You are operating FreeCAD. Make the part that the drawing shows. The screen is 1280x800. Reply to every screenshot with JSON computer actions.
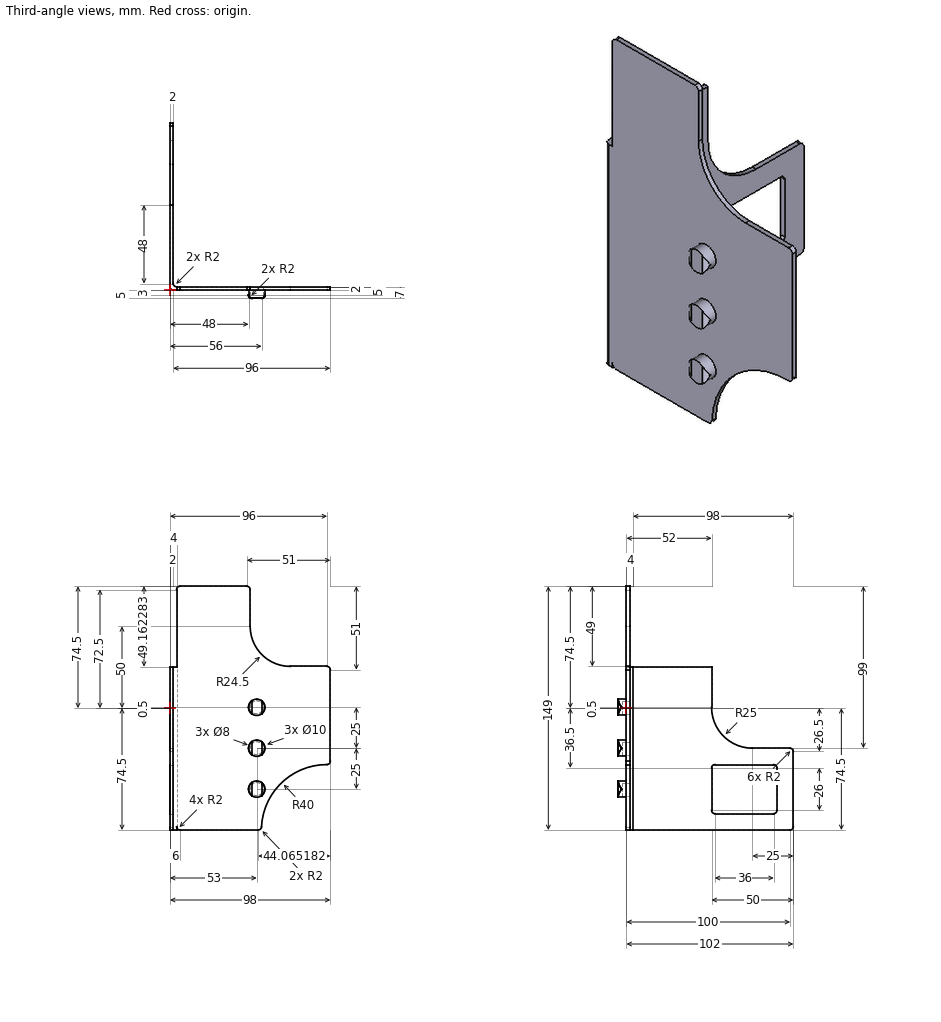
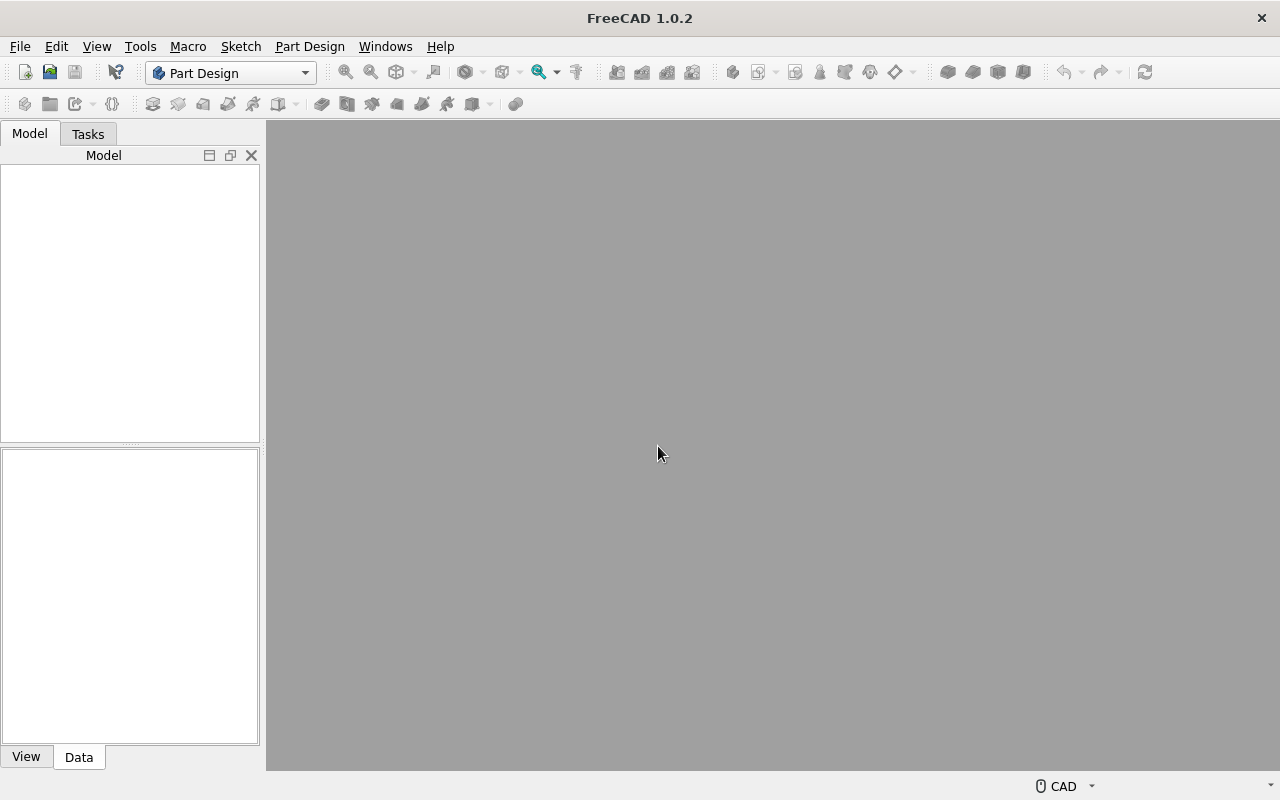
{"action": "key", "text": "ctrl+n"}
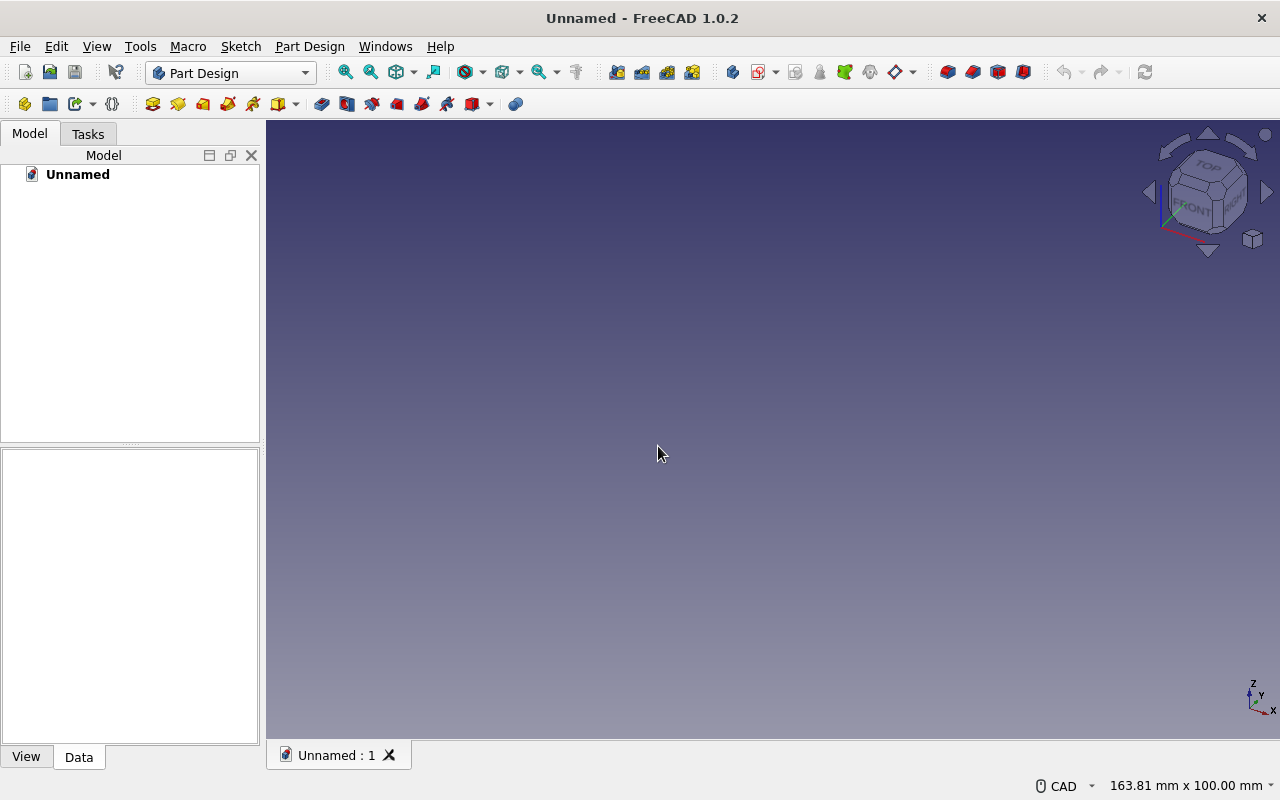
{"action": "left_click", "coordinate": [758, 72]}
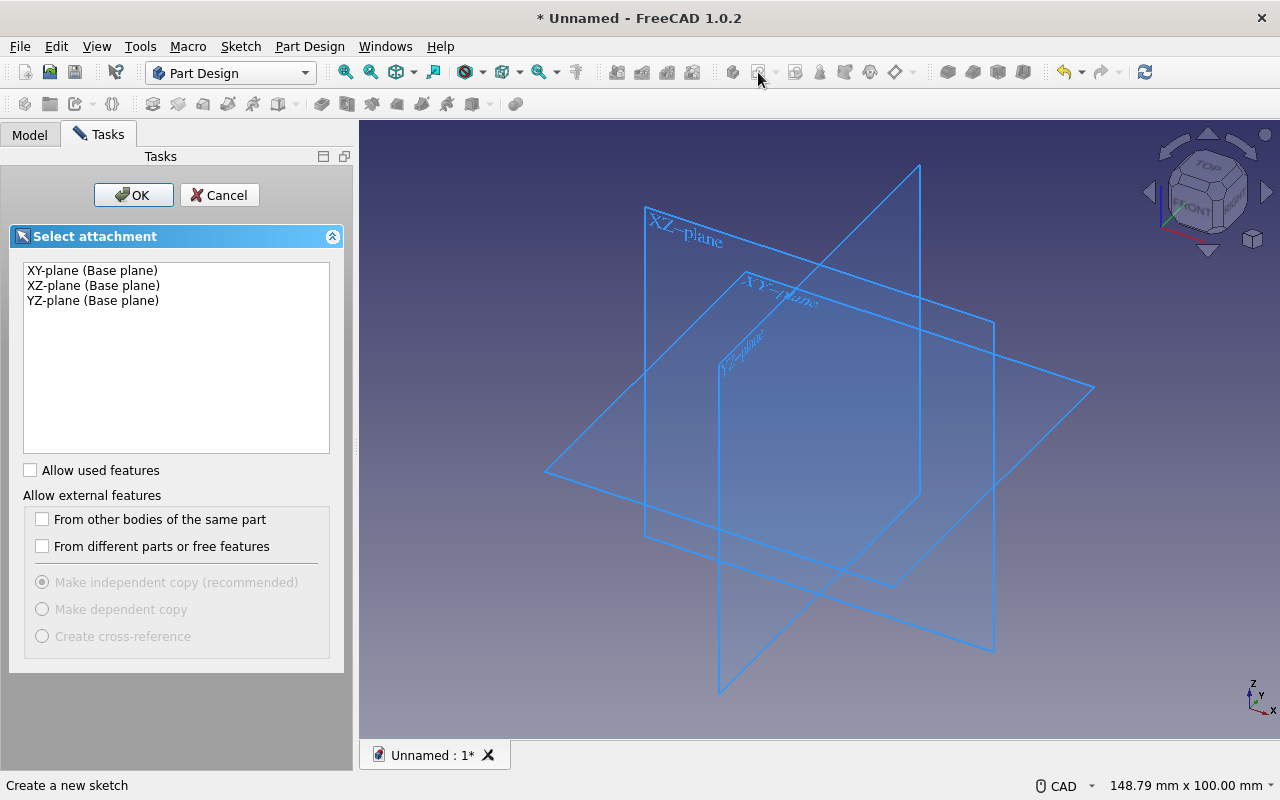
{"action": "left_click", "coordinate": [84, 270]}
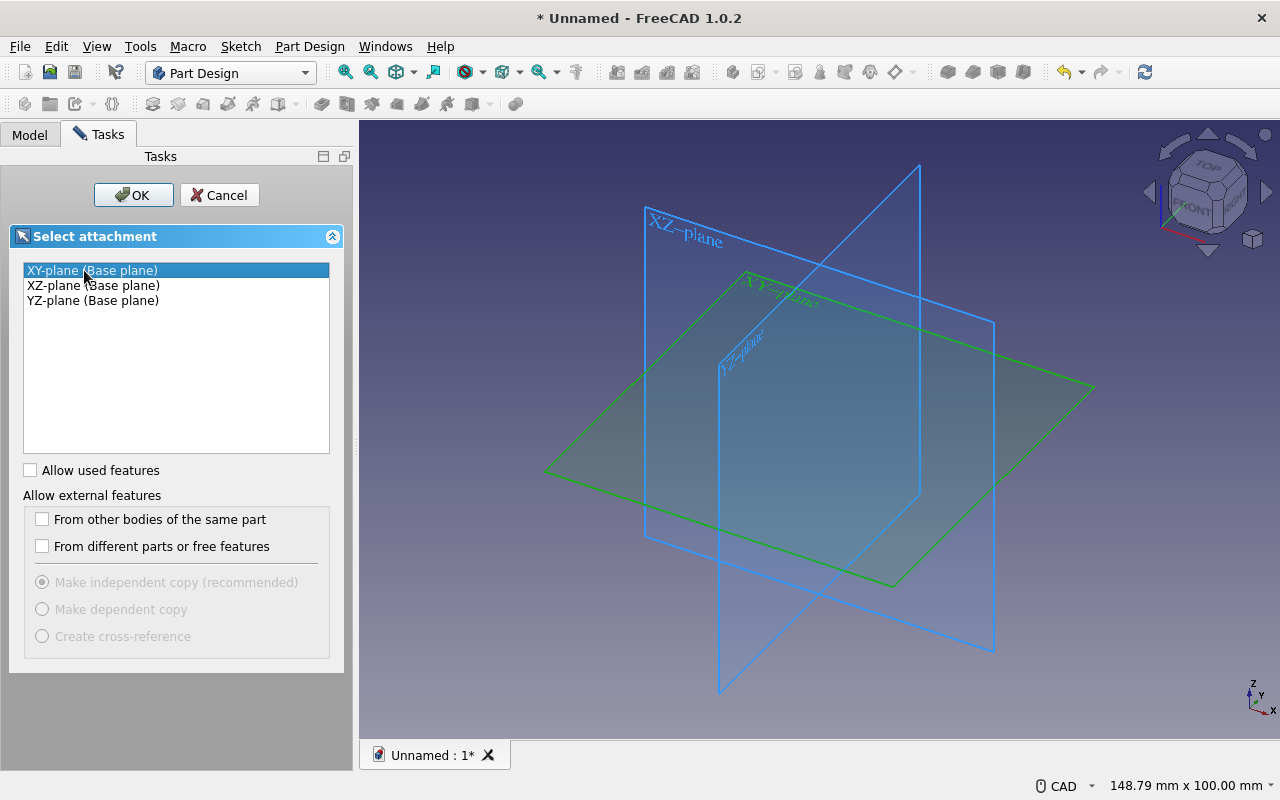
{"action": "left_click", "coordinate": [134, 195]}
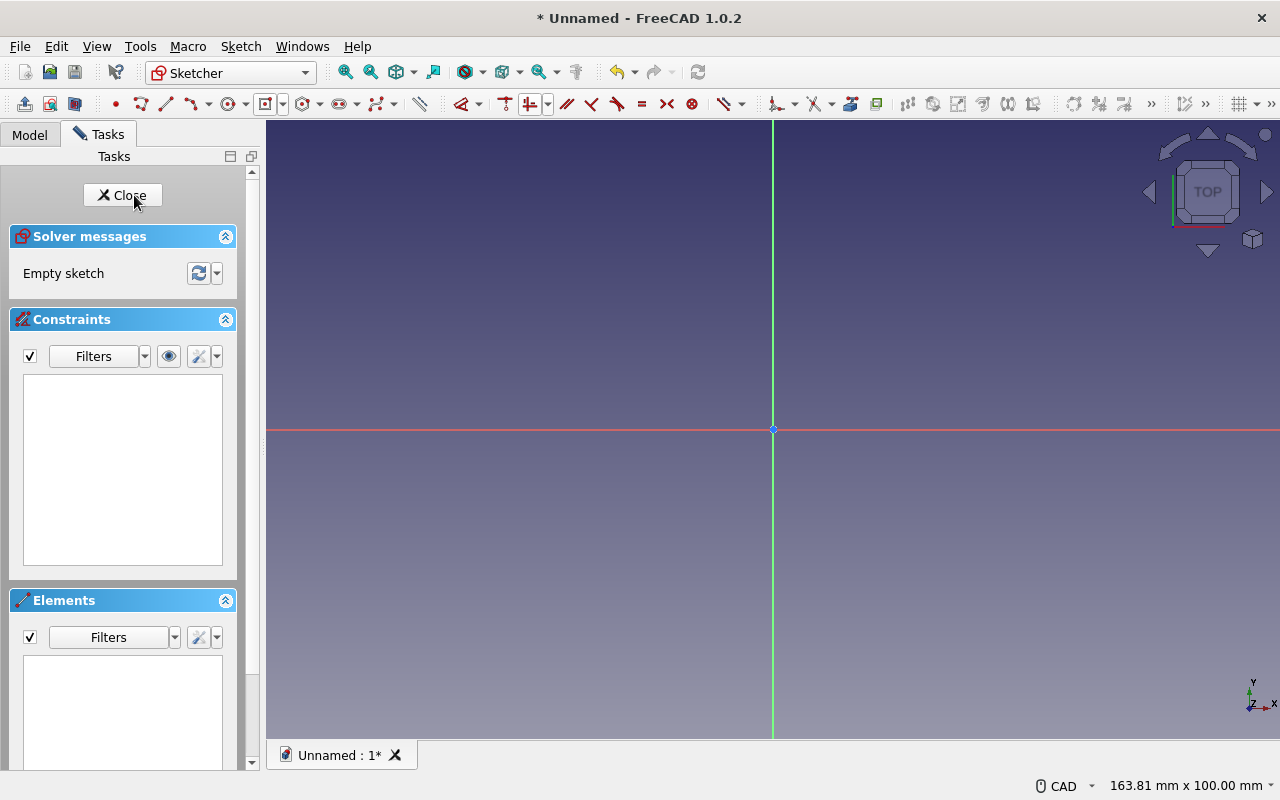
{"action": "scroll", "coordinate": [294, 711], "scroll_direction": "down", "scroll_amount": 2}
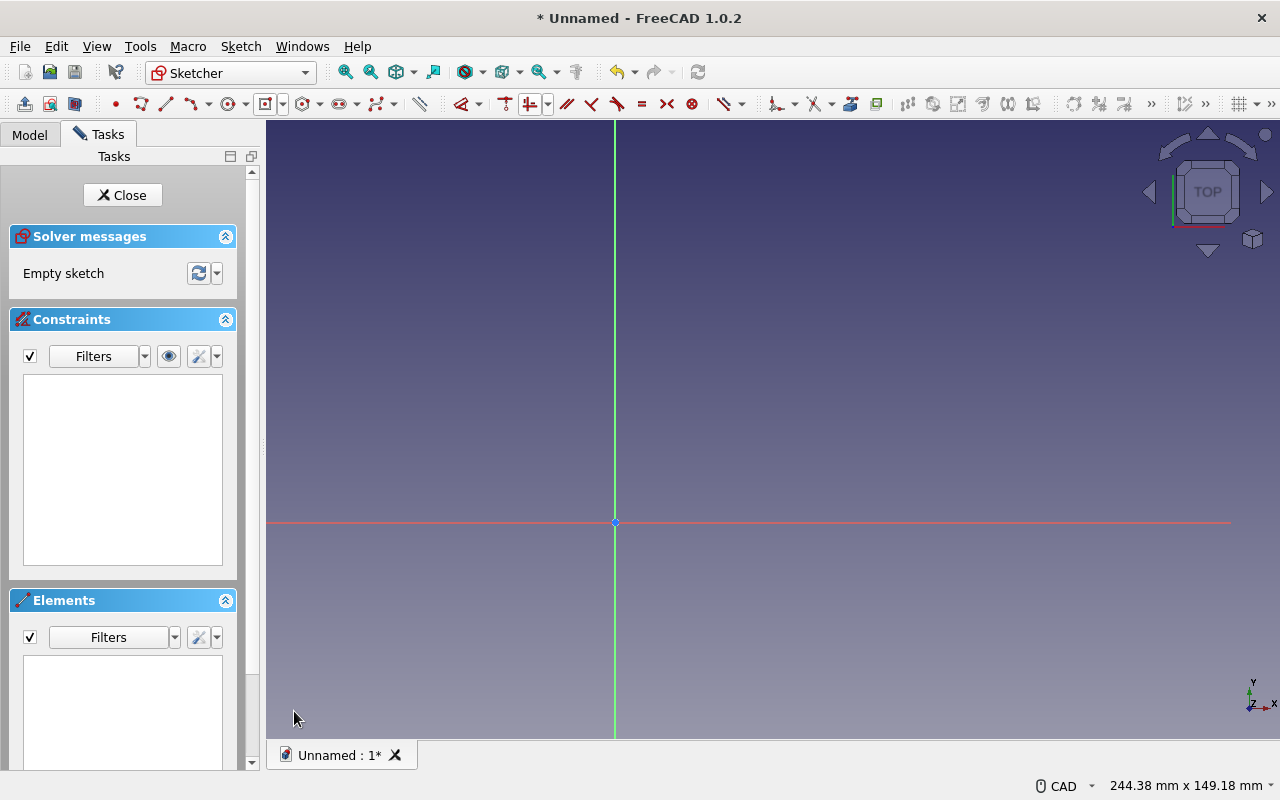
{"action": "scroll", "coordinate": [1050, 385], "scroll_direction": "up", "scroll_amount": 2}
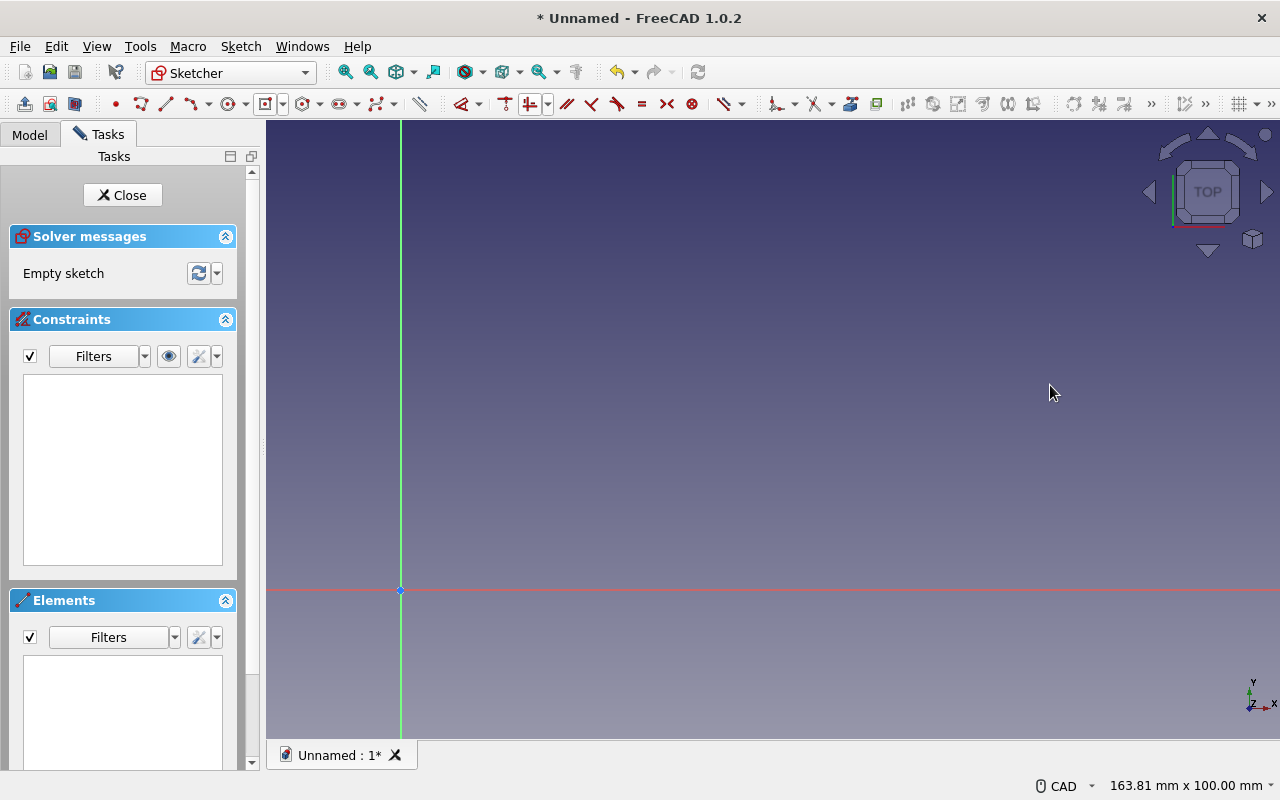
{"action": "key", "text": "g m"}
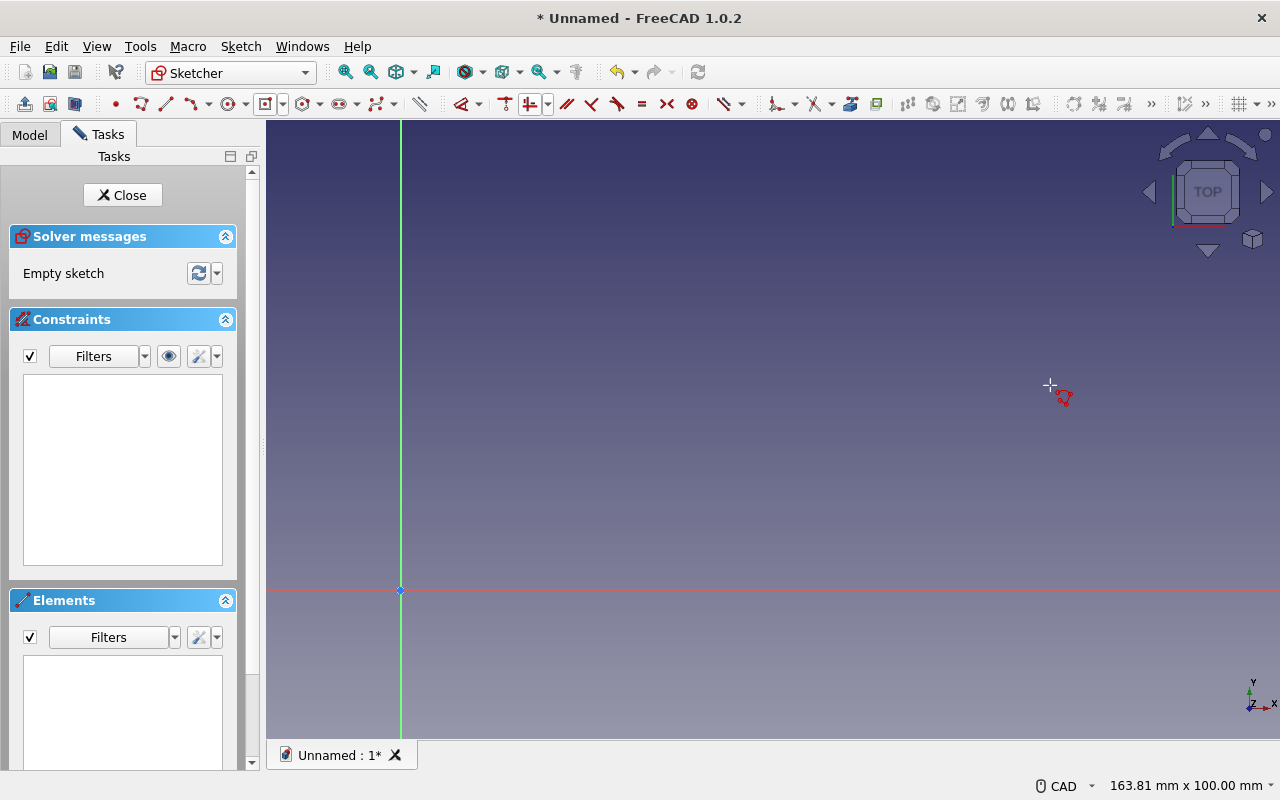
{"action": "scroll", "coordinate": [413, 590], "scroll_direction": "up", "scroll_amount": 2}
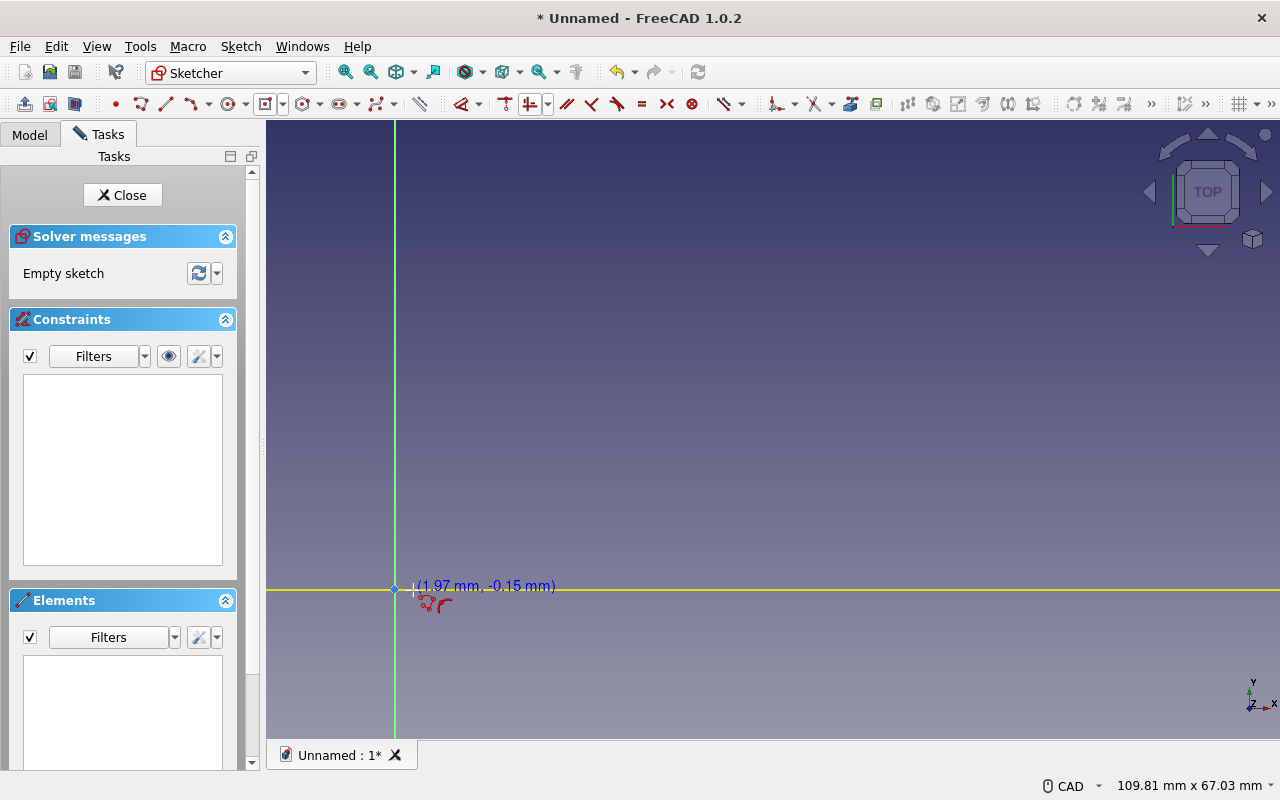
{"action": "left_click", "coordinate": [413, 590]}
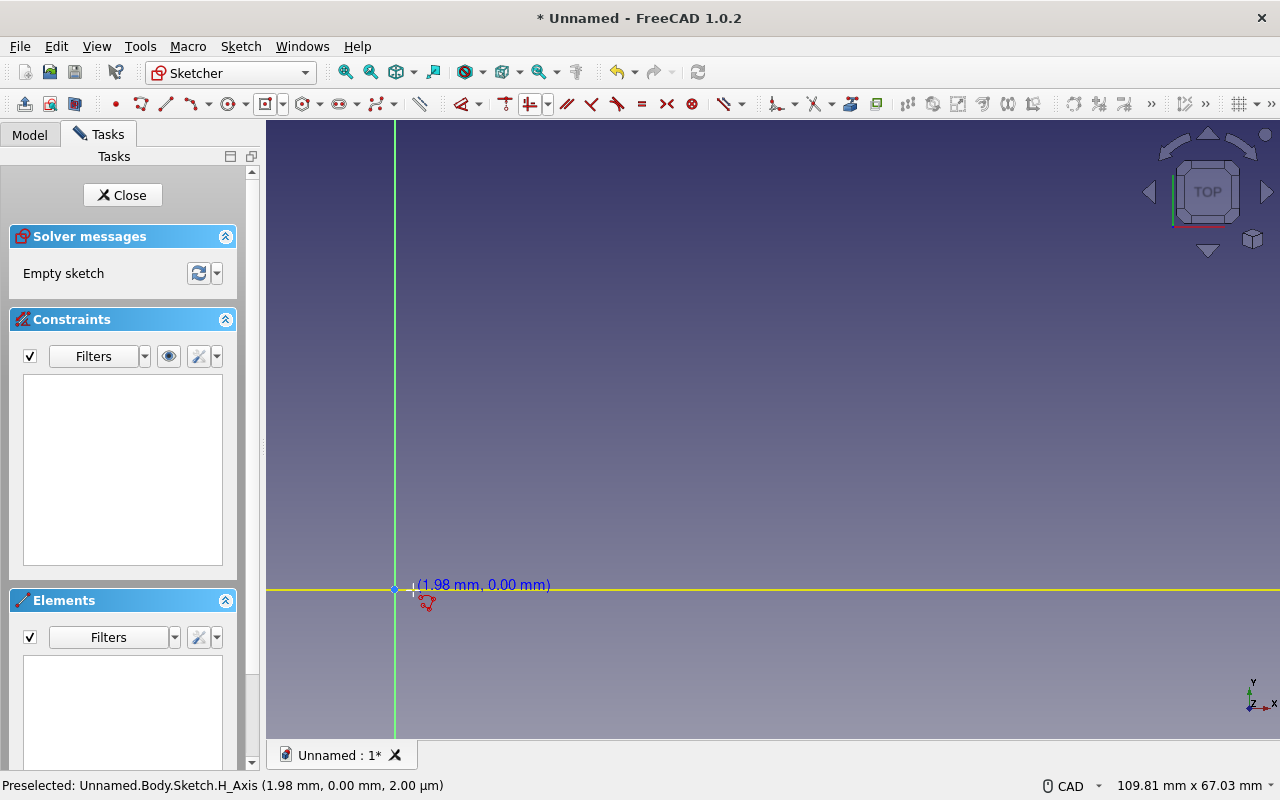
{"action": "scroll", "coordinate": [414, 592], "scroll_direction": "down", "scroll_amount": 2}